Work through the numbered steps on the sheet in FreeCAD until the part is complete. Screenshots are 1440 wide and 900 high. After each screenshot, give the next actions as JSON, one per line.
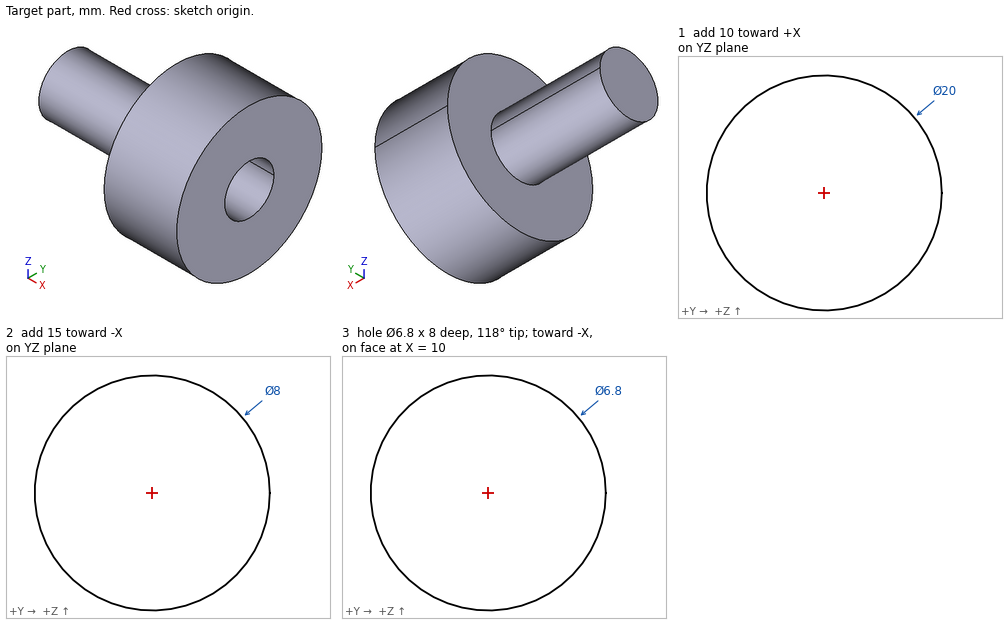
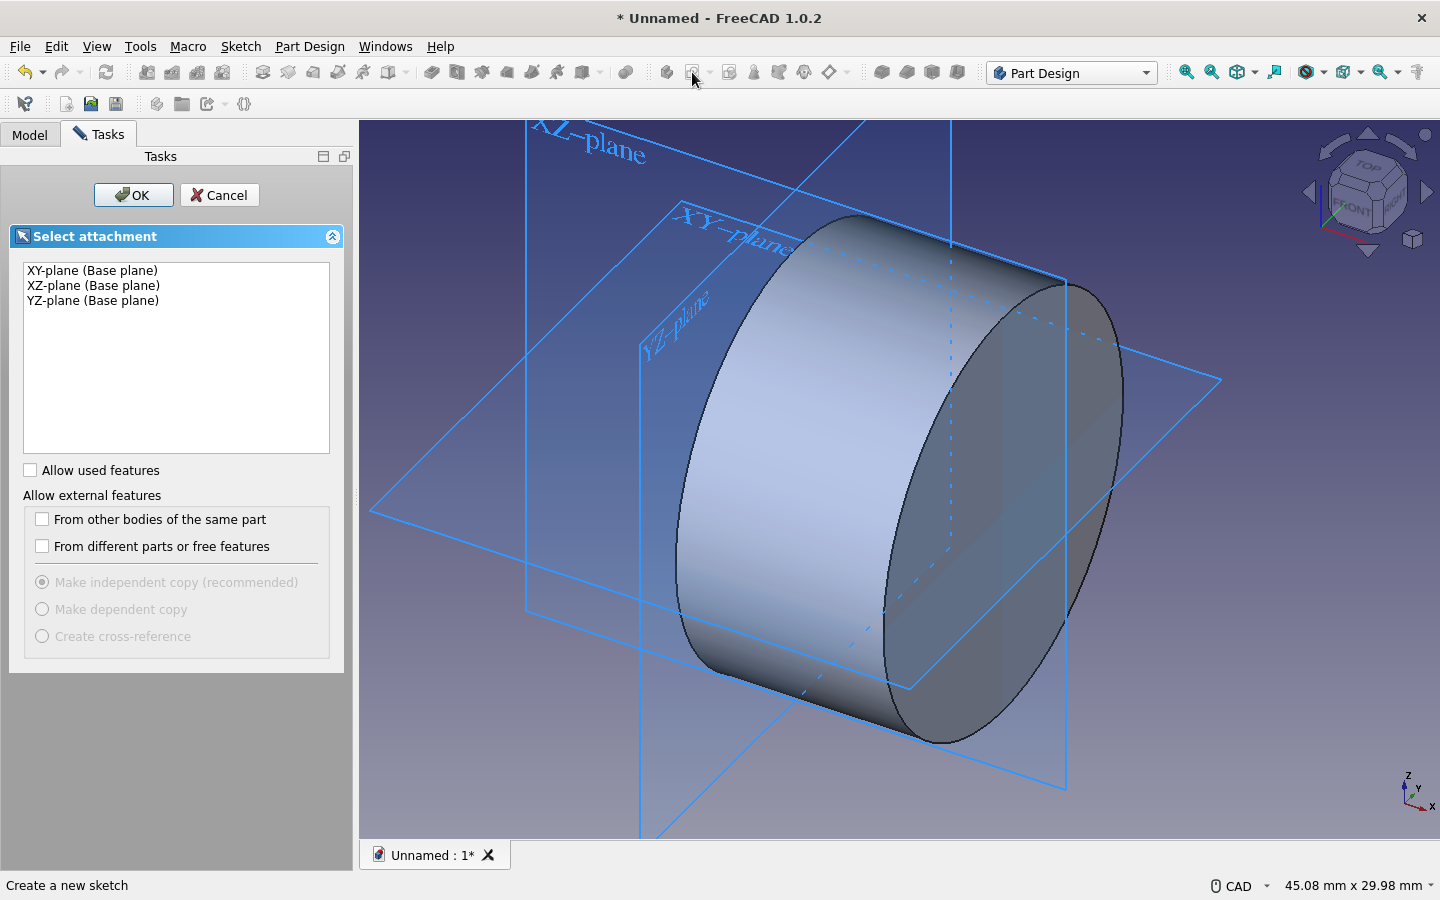
{"action": "left_click", "coordinate": [84, 300]}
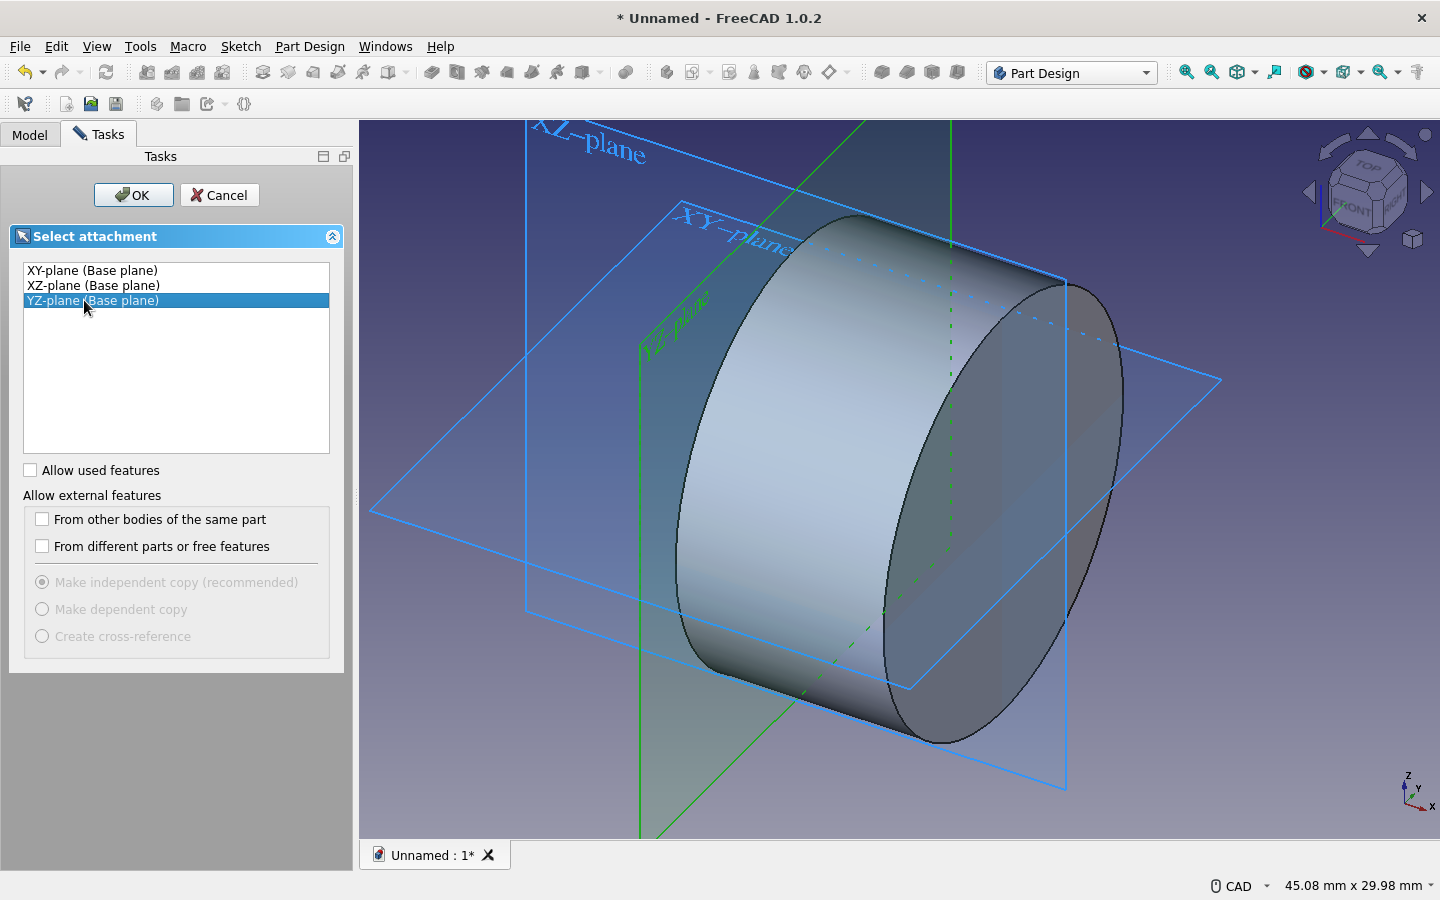
{"action": "left_click", "coordinate": [134, 195]}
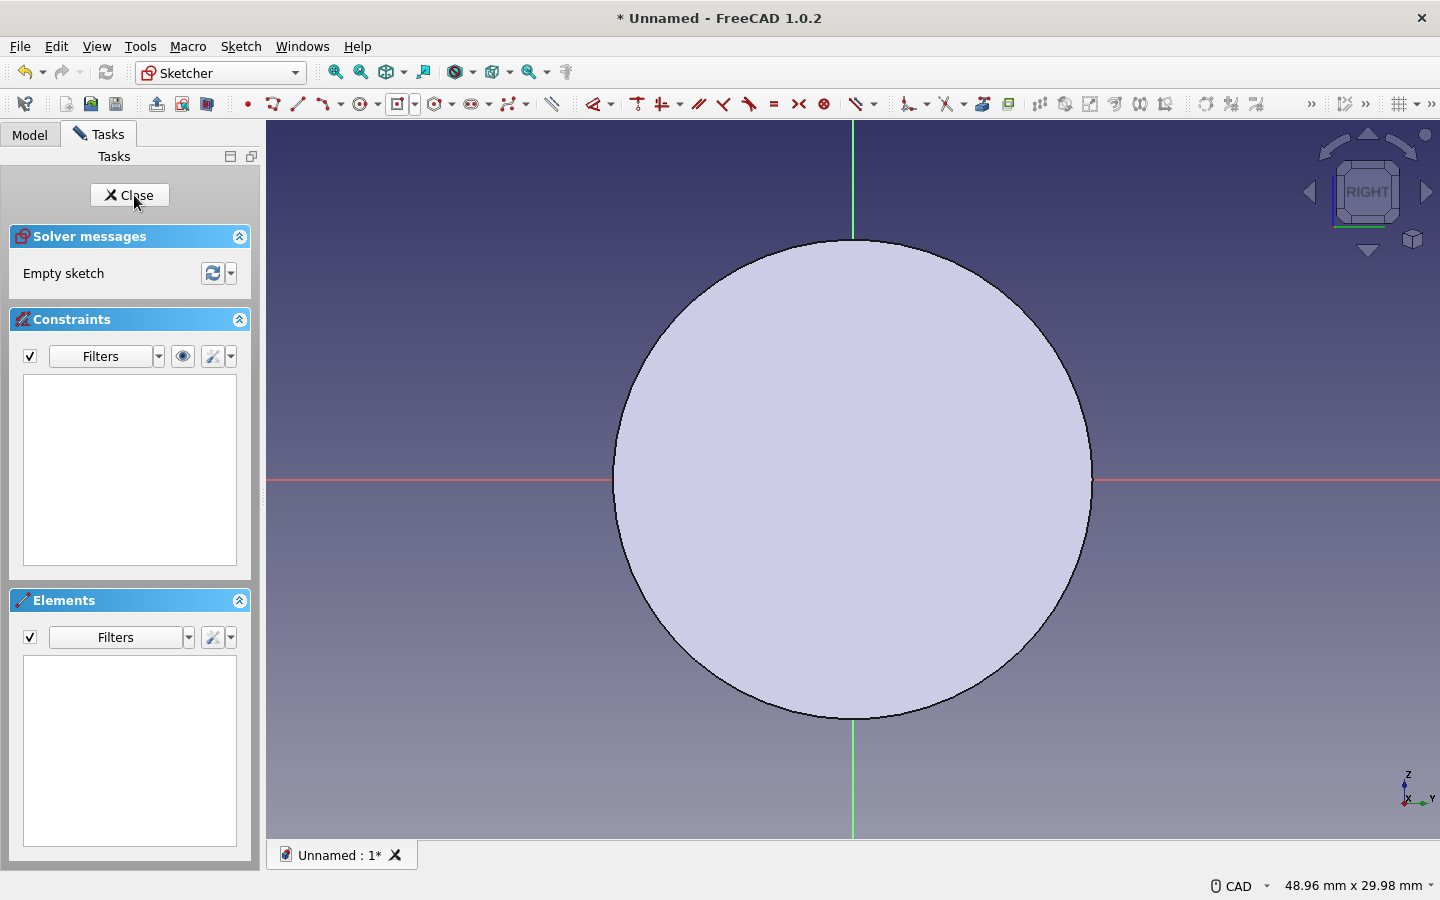
{"action": "left_click", "coordinate": [207, 104]}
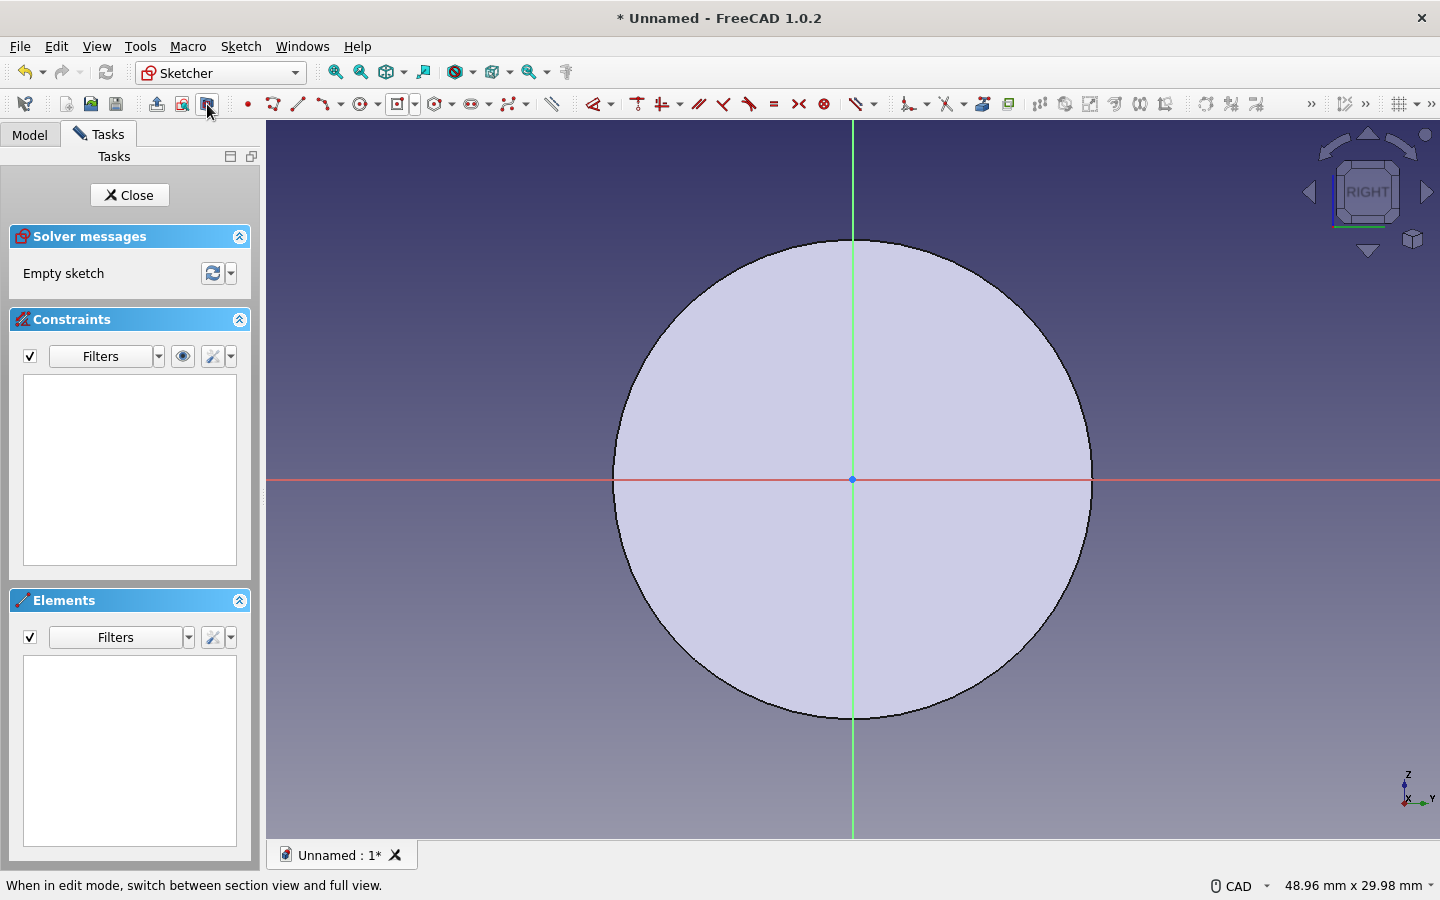
{"action": "scroll", "coordinate": [909, 480], "scroll_direction": "up", "scroll_amount": 4}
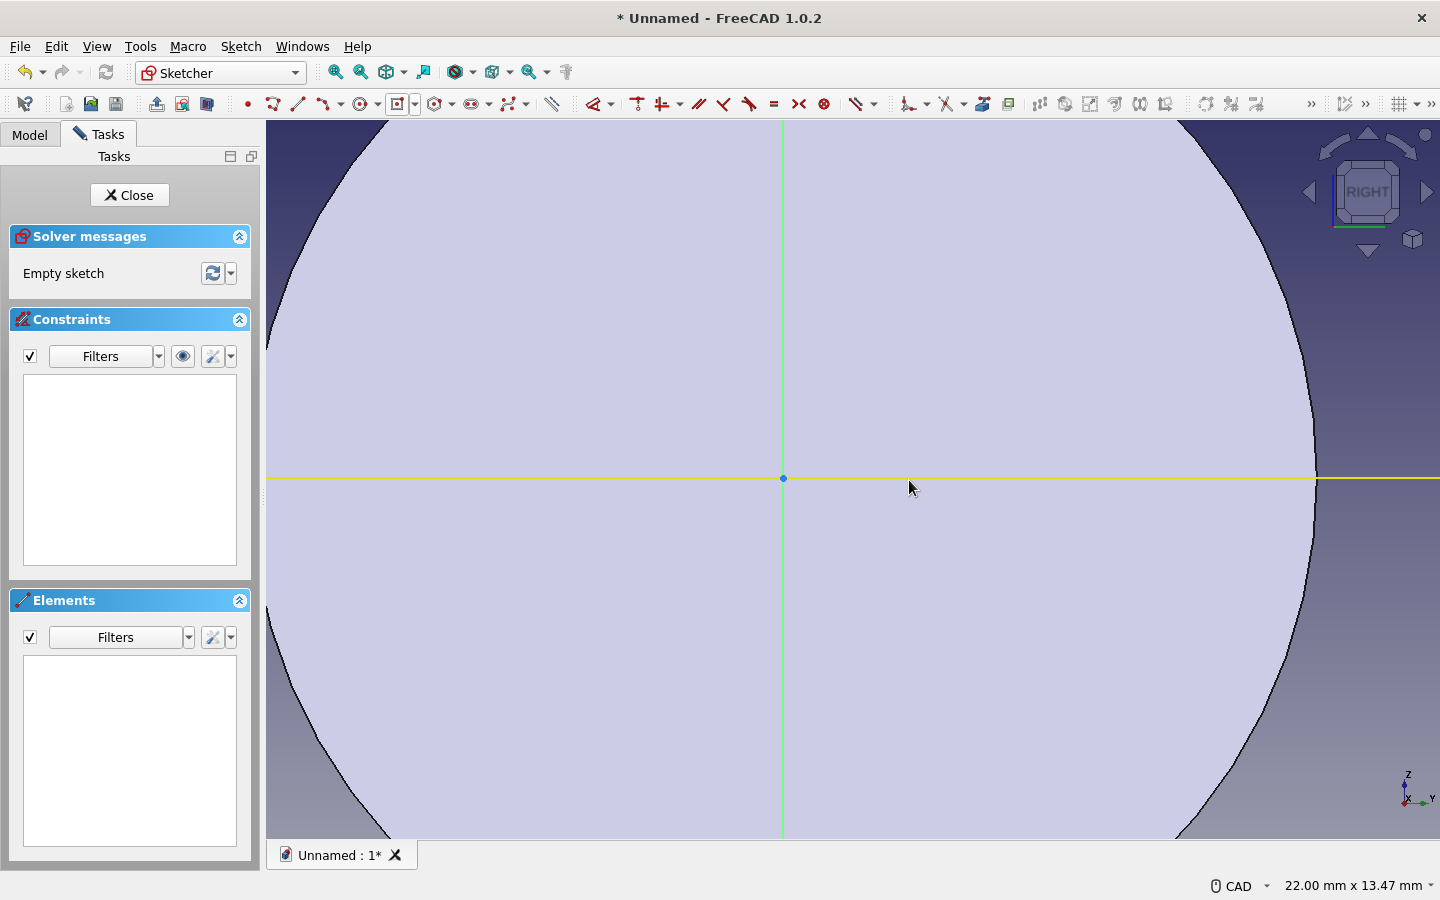
{"action": "left_click", "coordinate": [360, 104]}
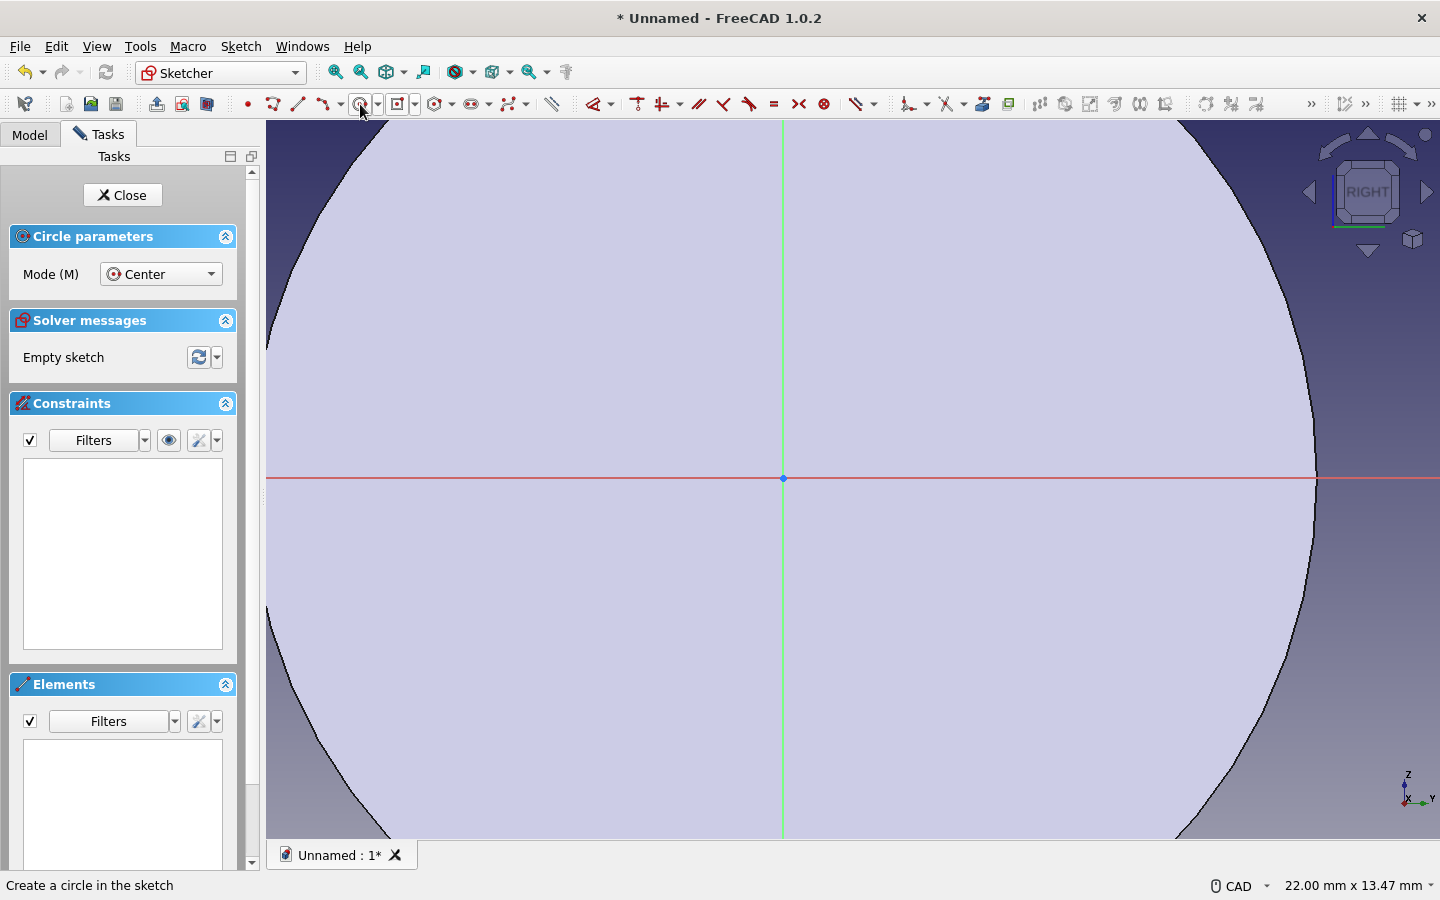
{"action": "left_click", "coordinate": [783, 478]}
{"action": "left_click", "coordinate": [934, 327]}
{"action": "key", "text": "Escape"}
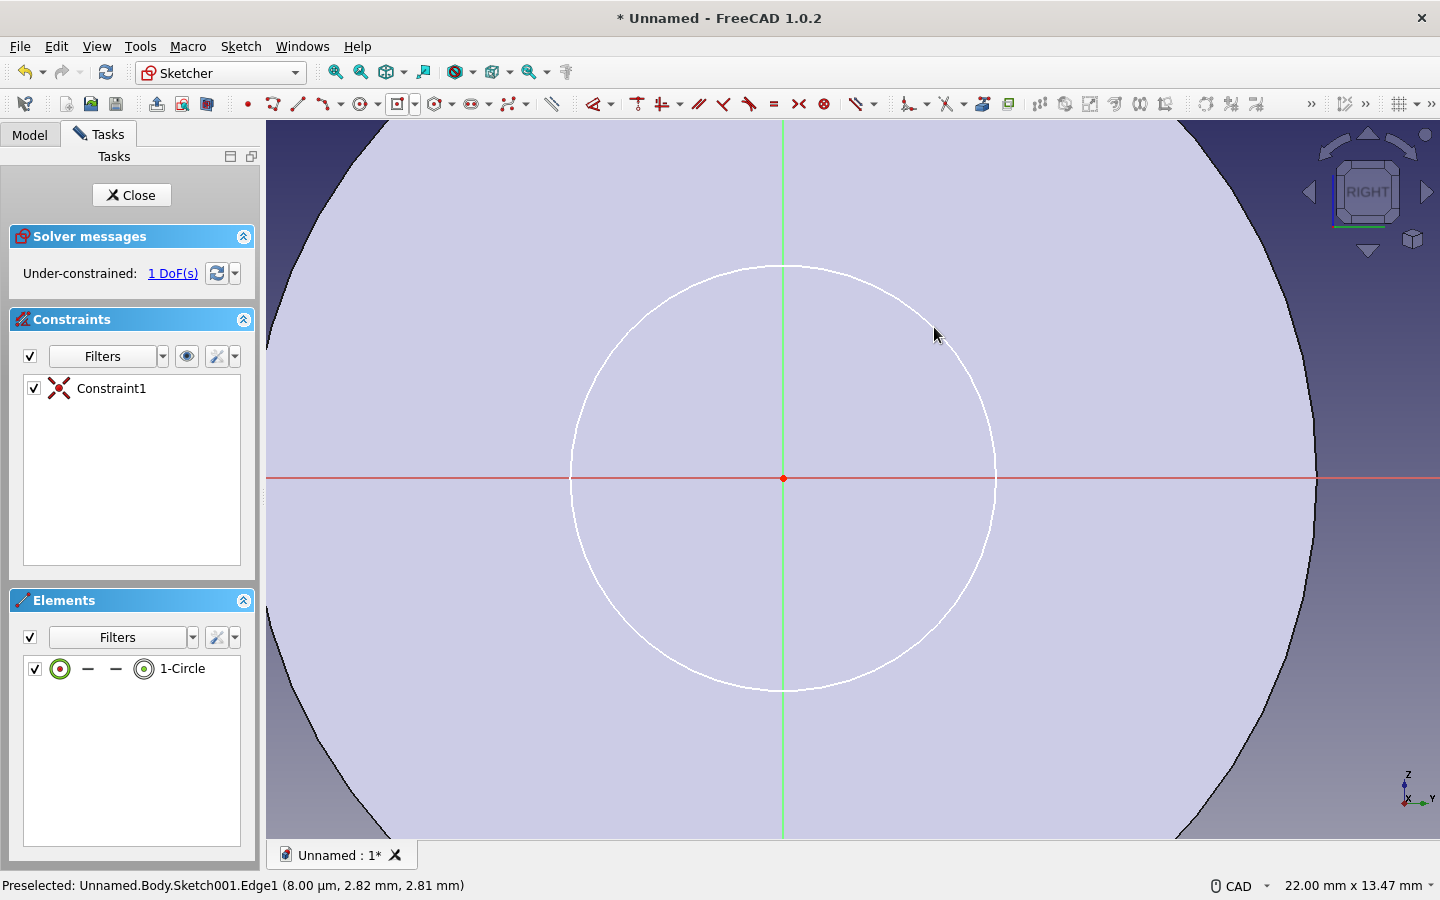
{"action": "left_click", "coordinate": [592, 104]}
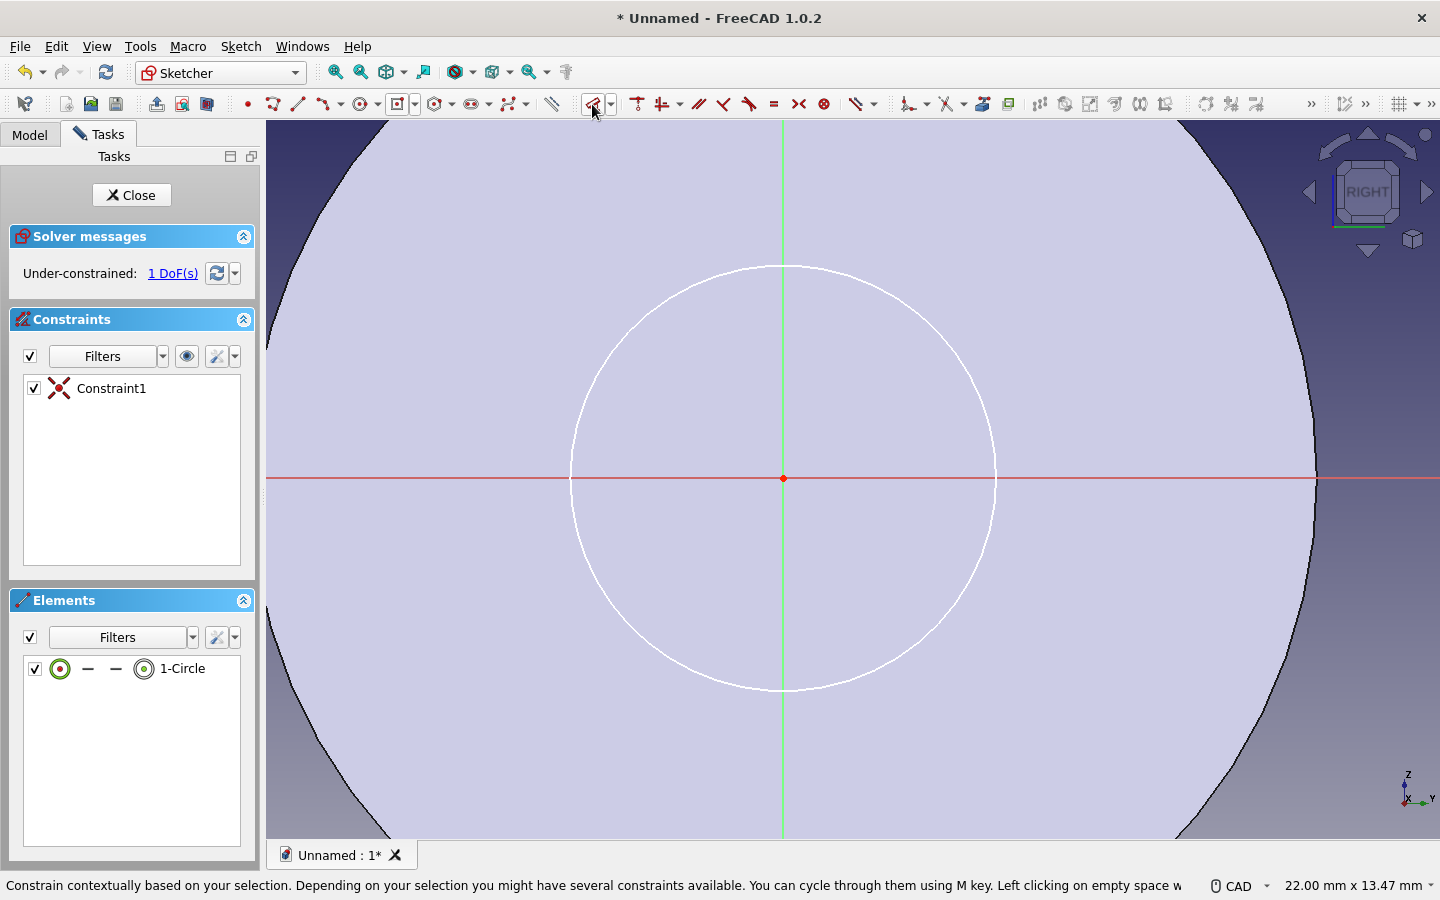
{"action": "left_click", "coordinate": [933, 327]}
{"action": "left_click", "coordinate": [956, 304]}